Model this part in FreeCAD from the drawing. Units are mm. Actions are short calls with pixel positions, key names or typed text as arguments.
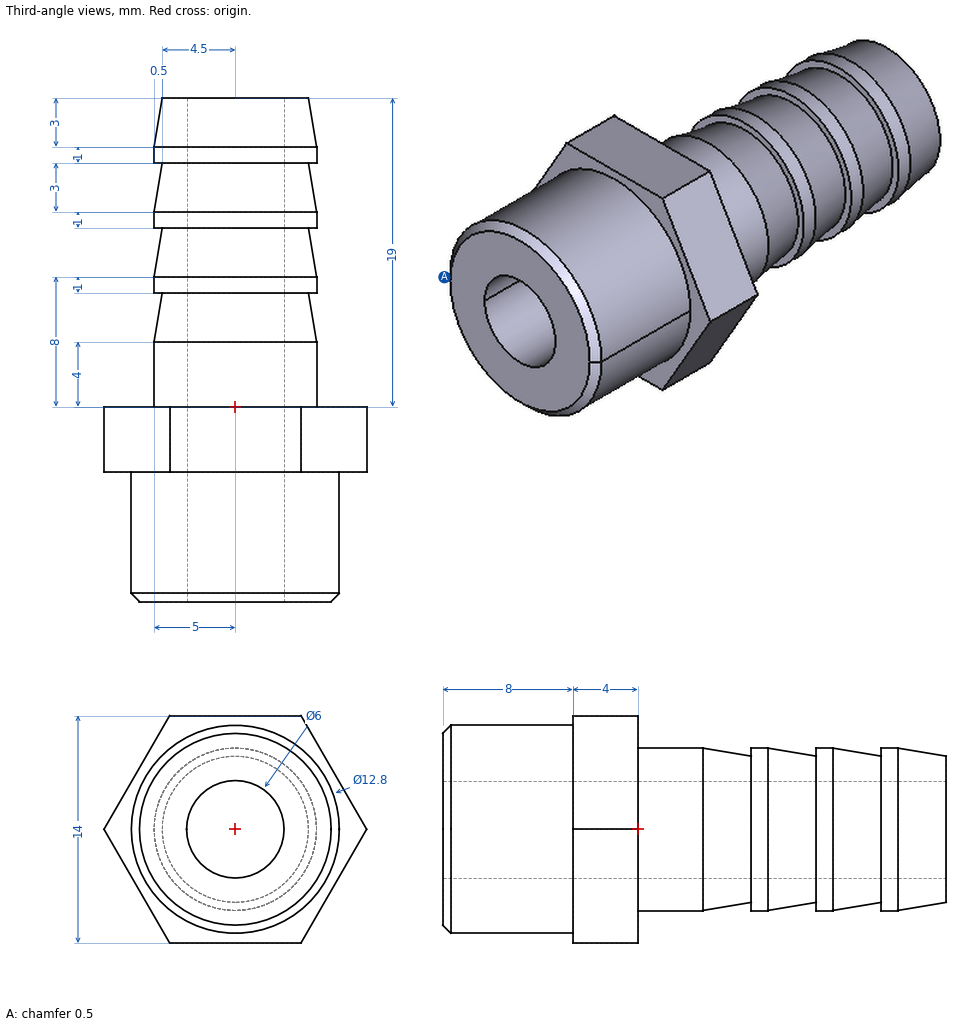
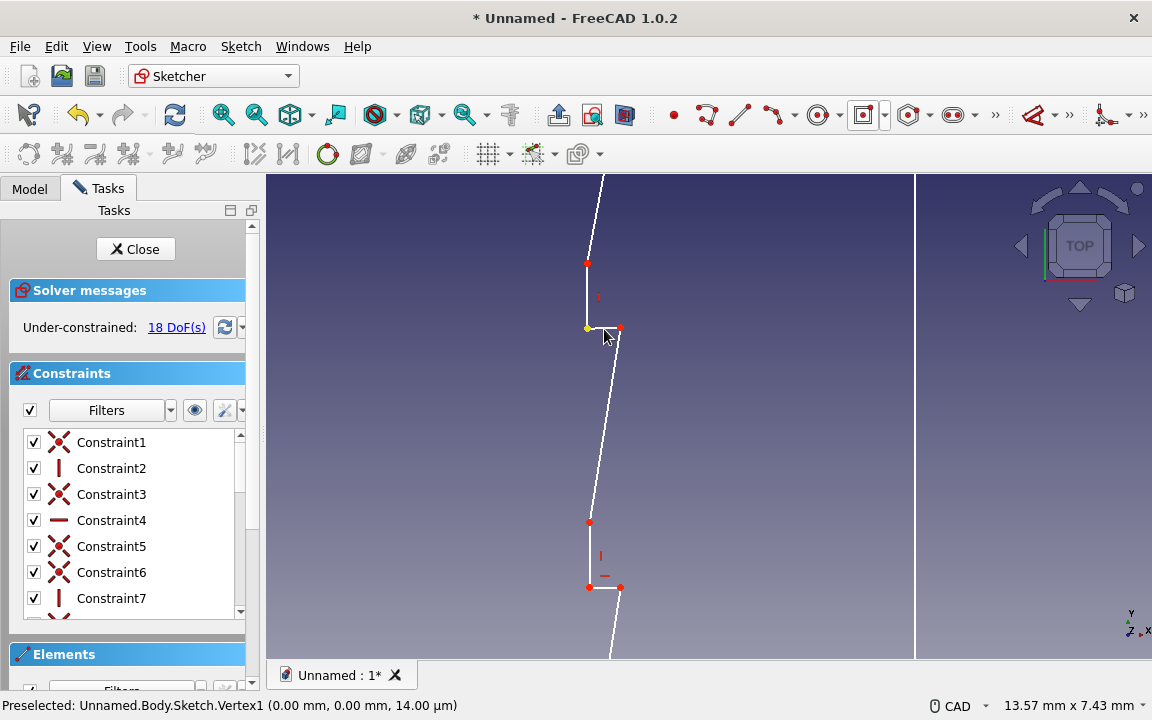
click(604, 328)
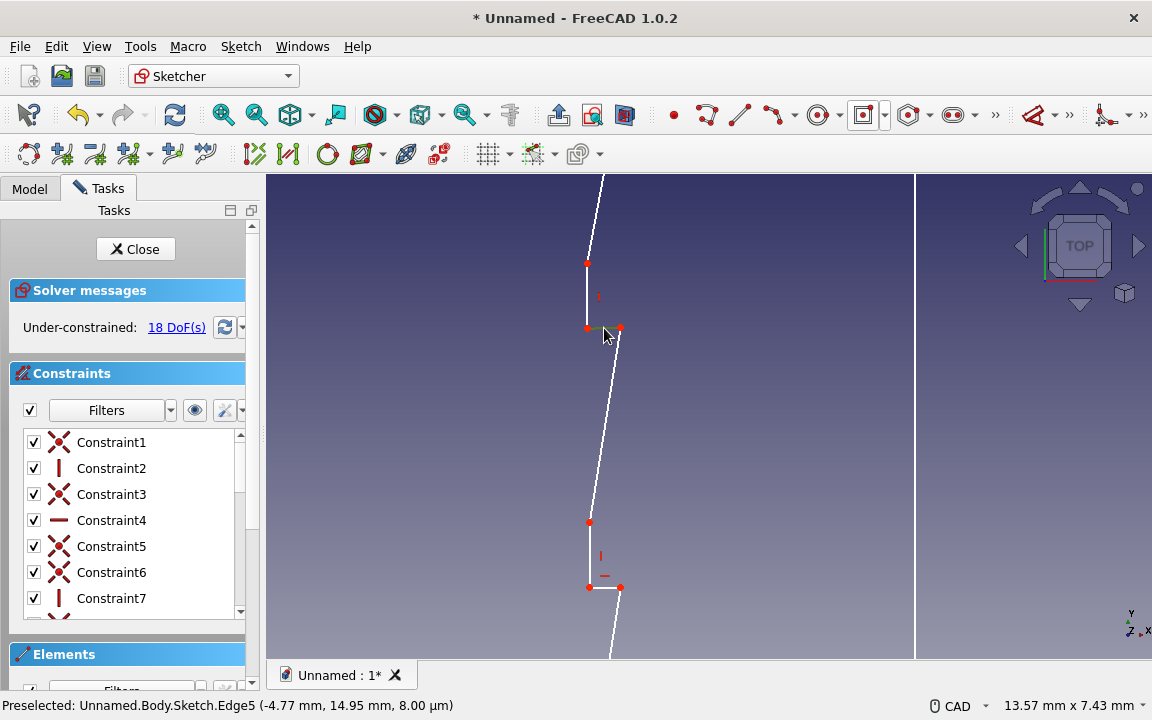
key(h)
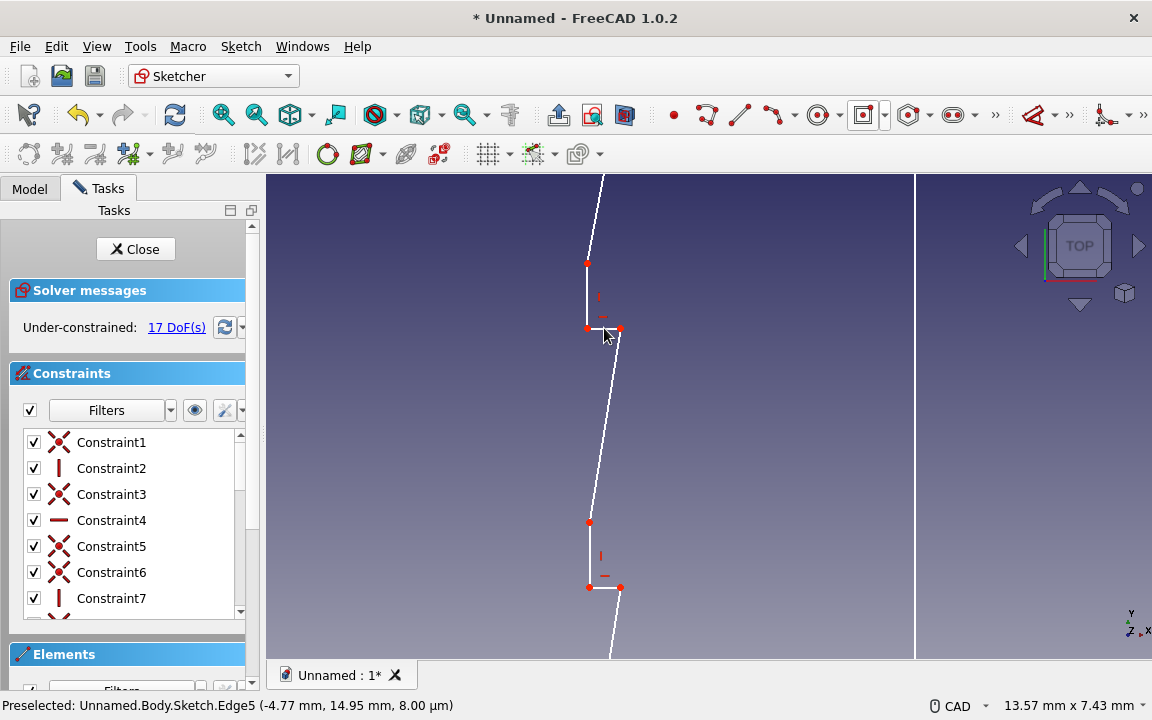
scroll(604, 329, down, 7)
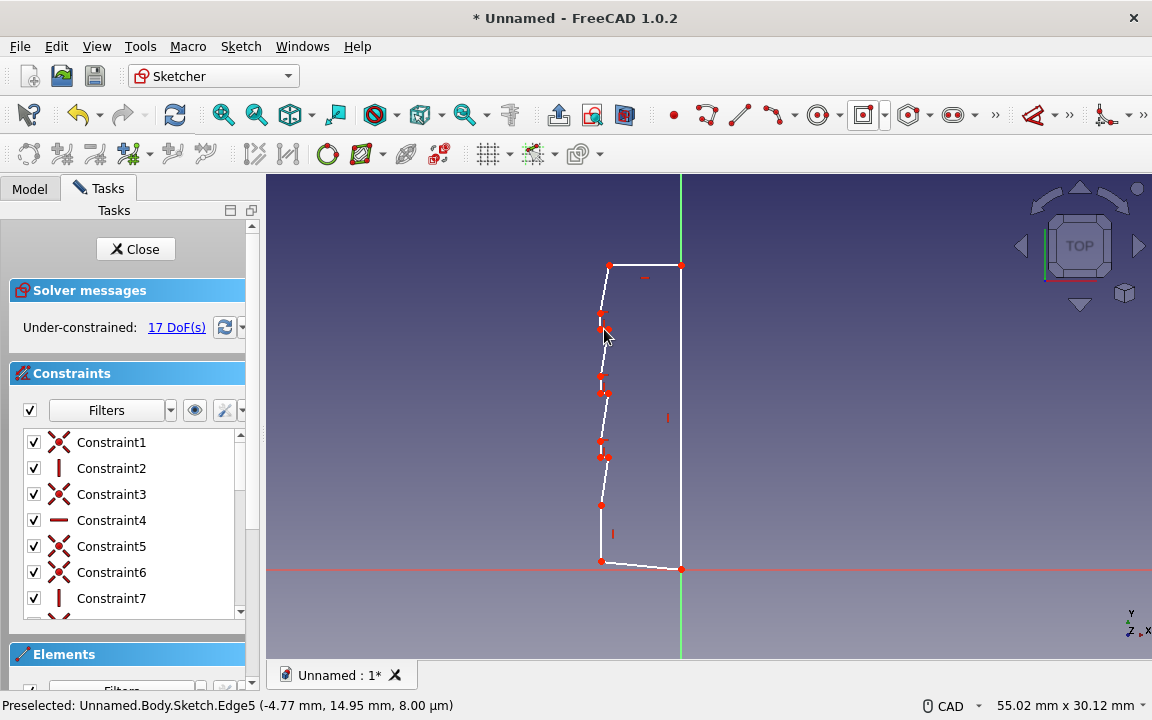
scroll(625, 564, up, 5)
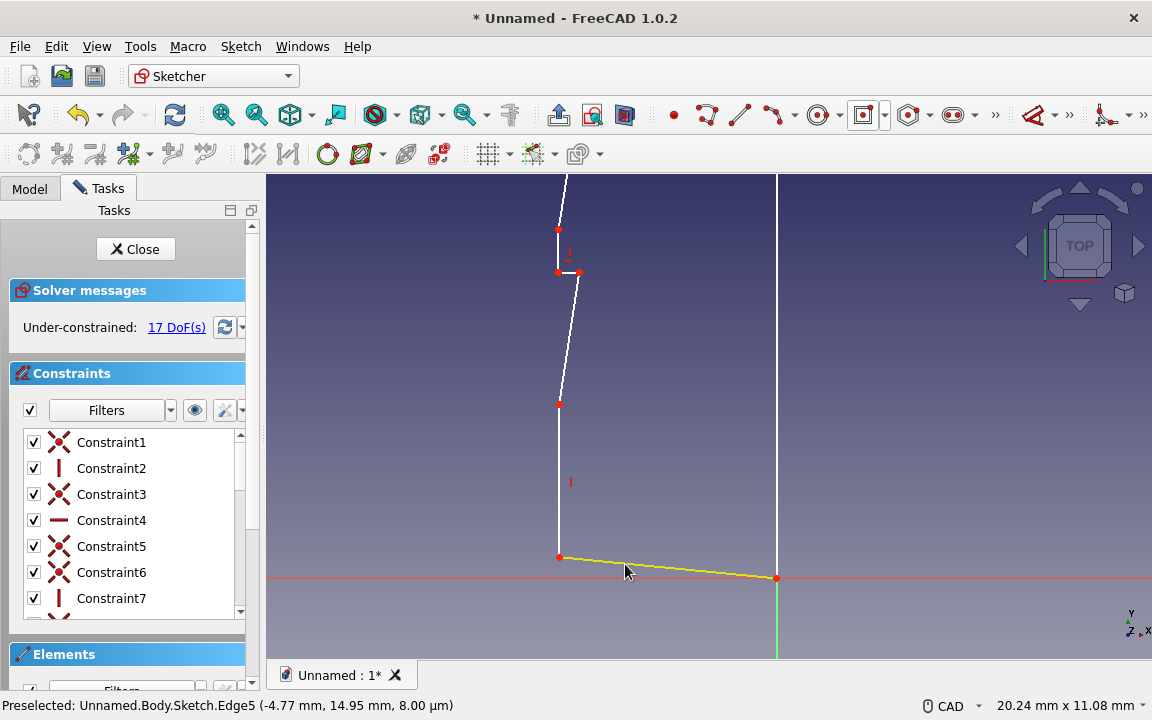
click(624, 564)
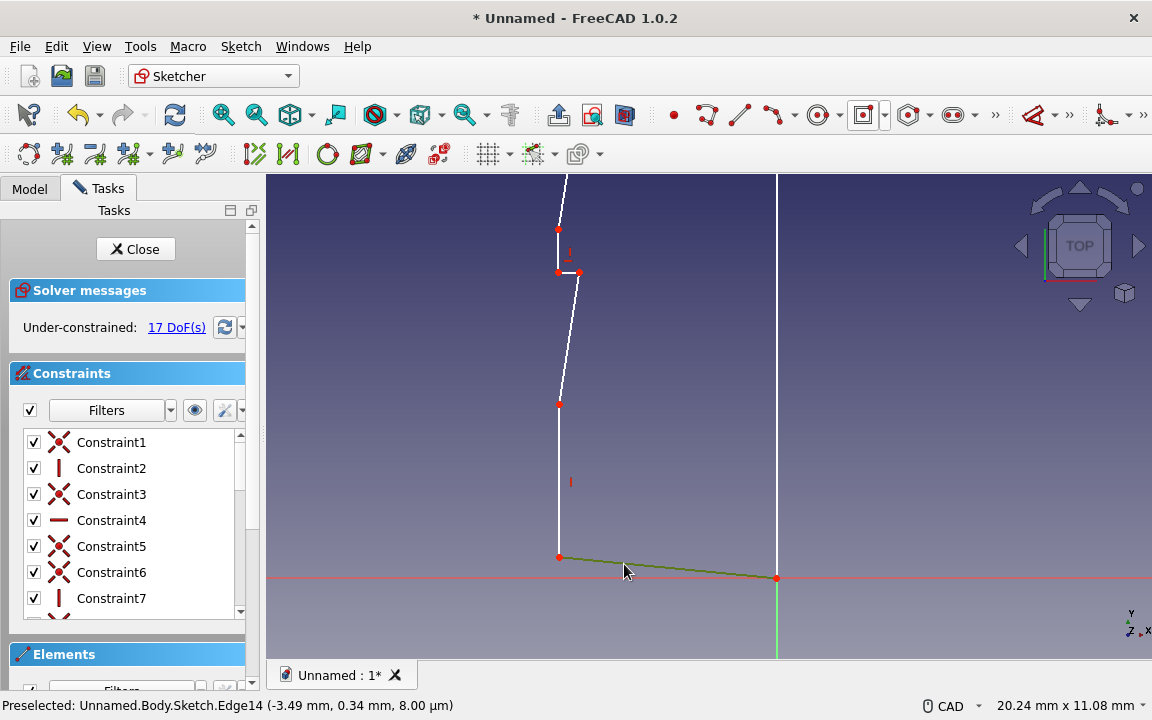
key(h)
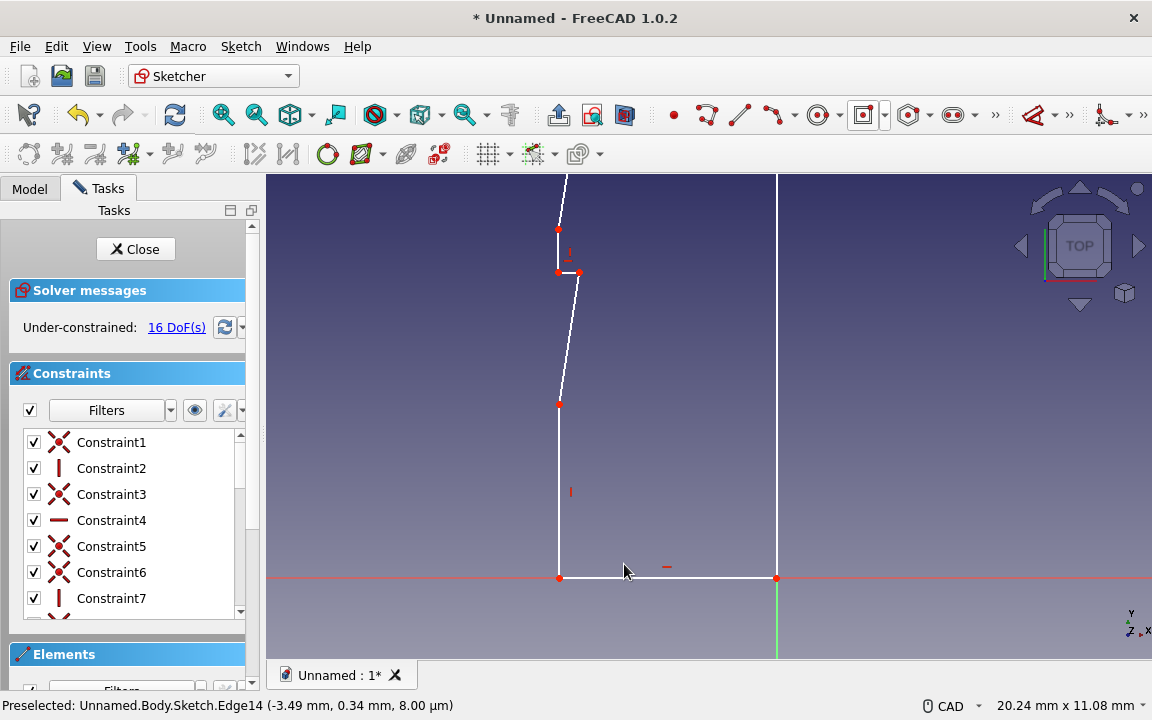
click(1032, 116)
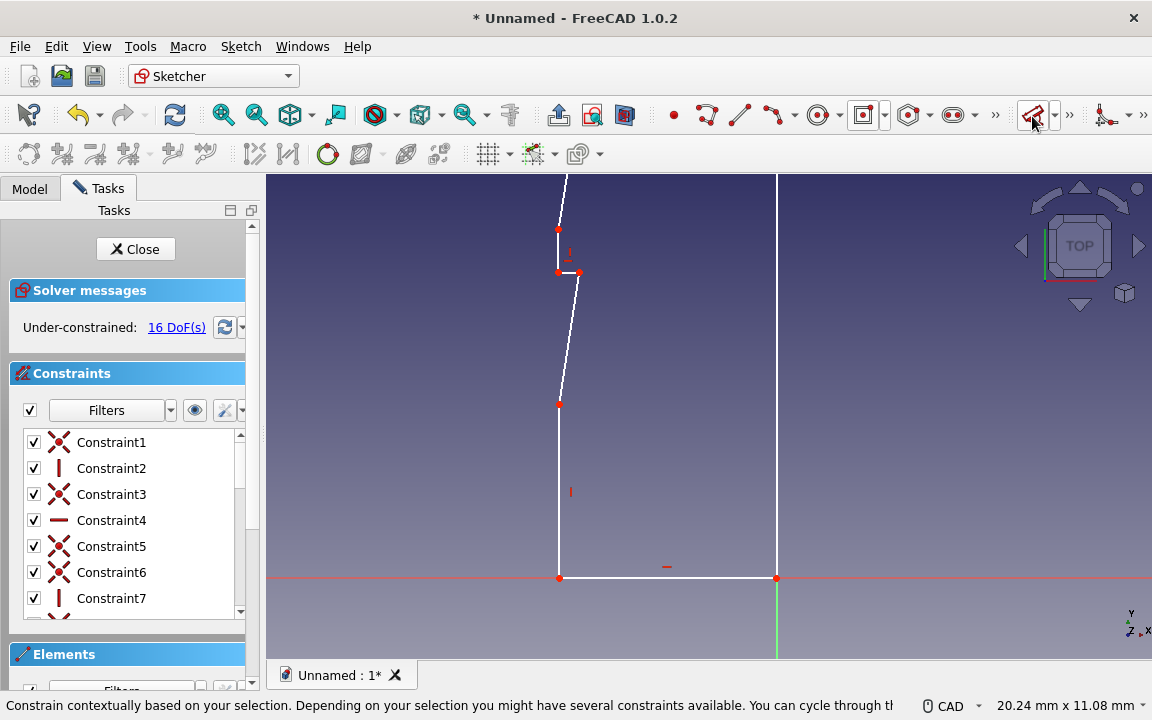
scroll(625, 564, down, 5)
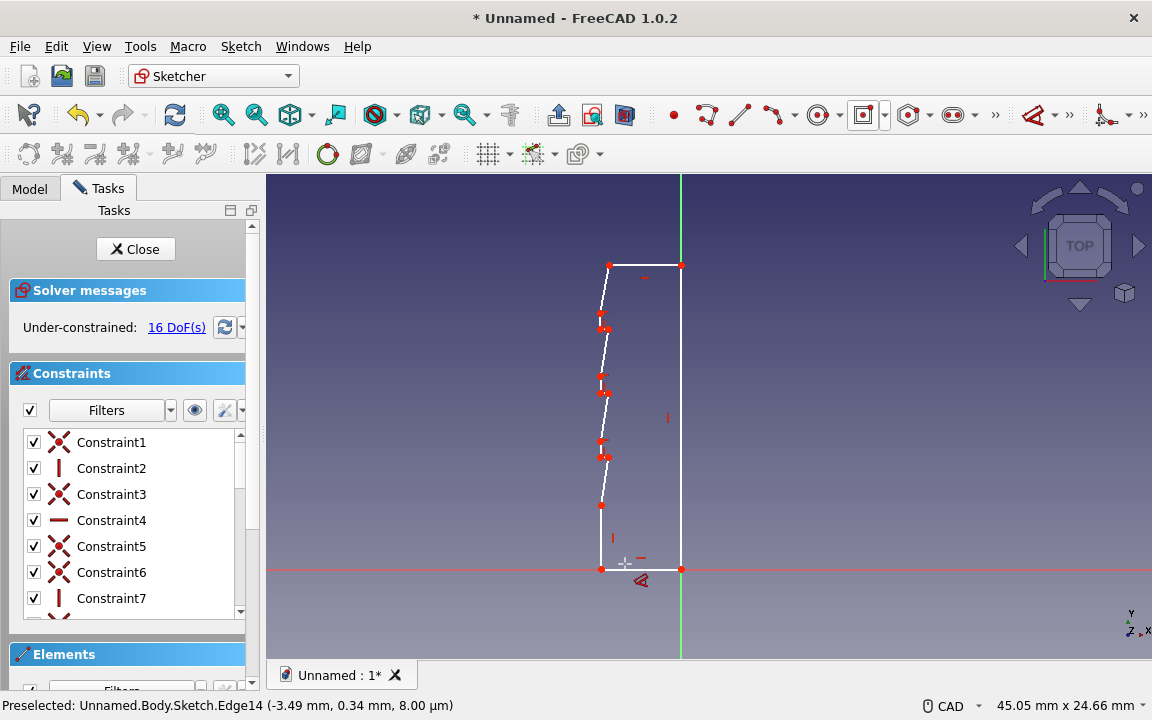
scroll(600, 318, up, 6)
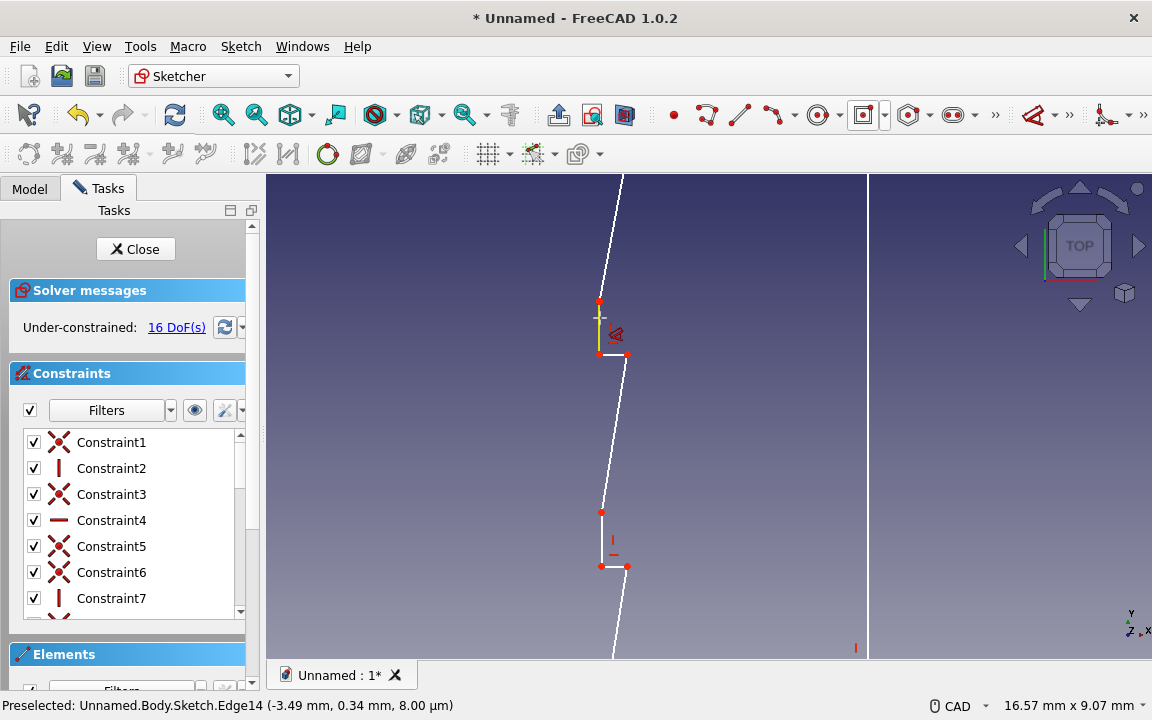
click(599, 317)
click(565, 328)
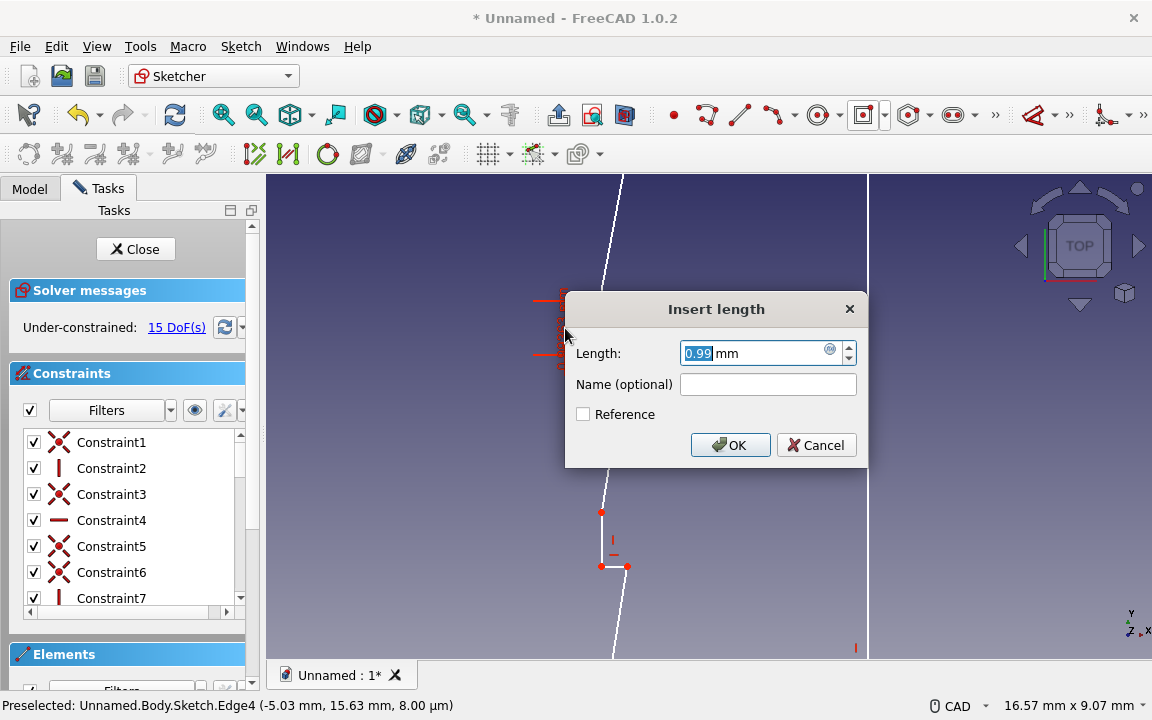
text(1)
key(Return)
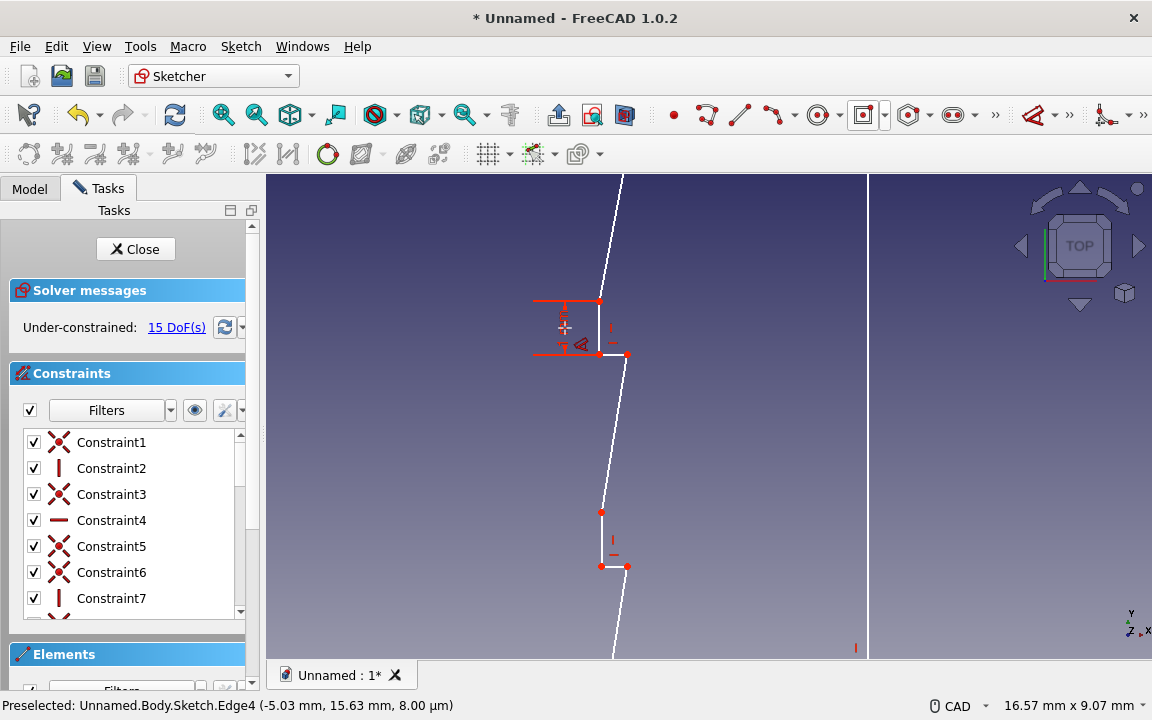
click(602, 529)
click(568, 540)